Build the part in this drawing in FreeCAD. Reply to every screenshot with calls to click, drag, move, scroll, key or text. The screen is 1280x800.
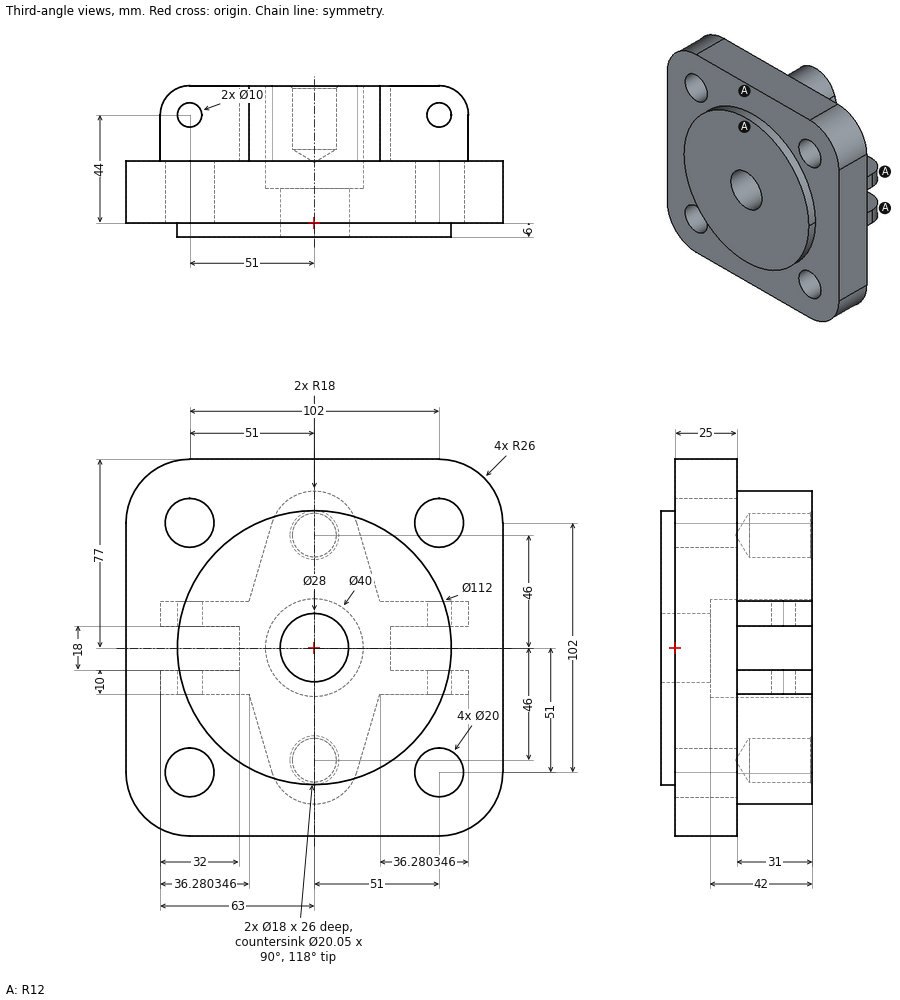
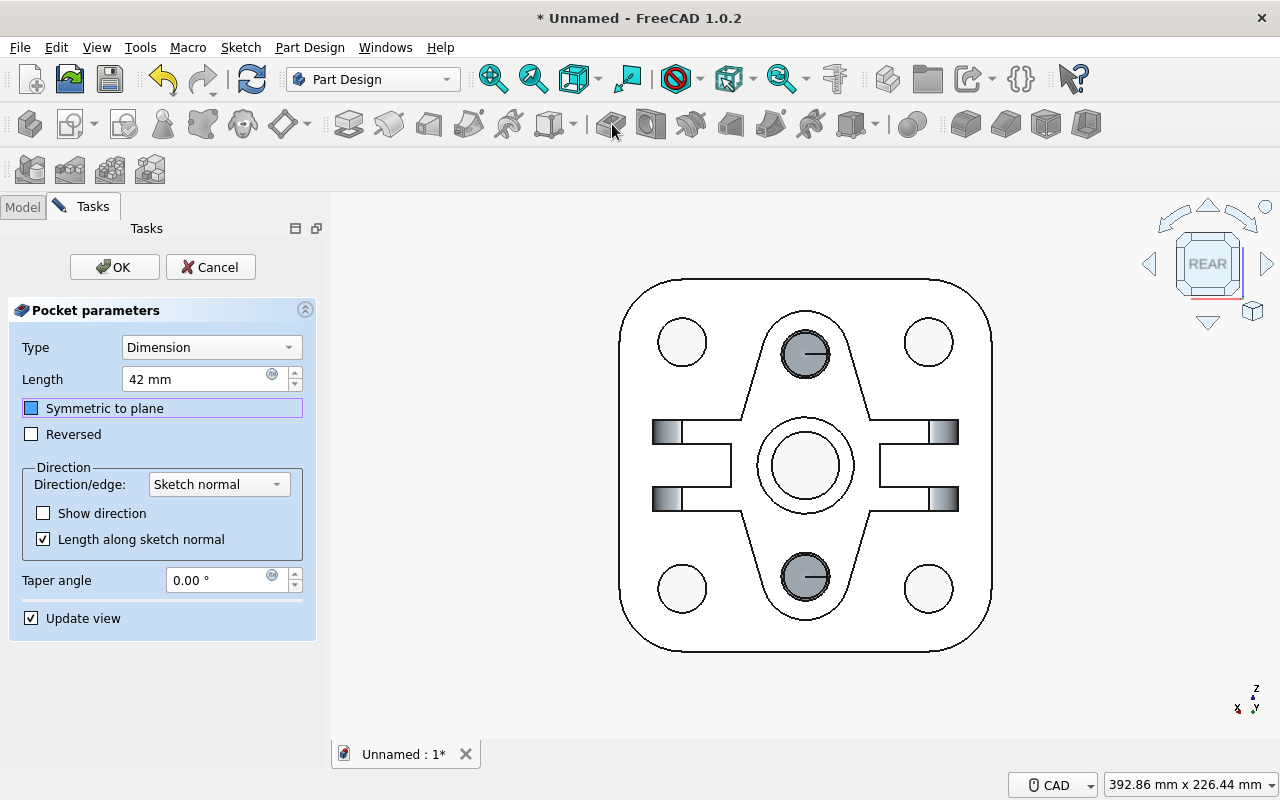
click(115, 267)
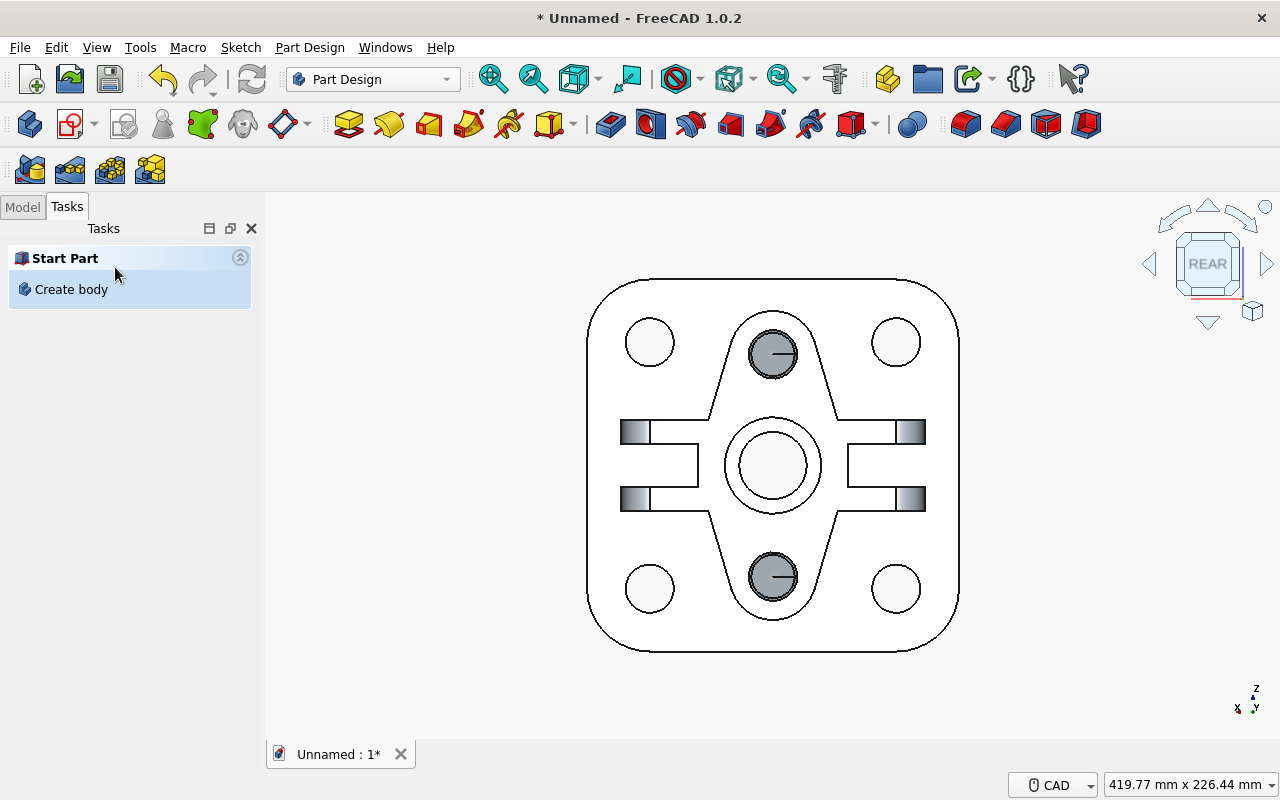
key(0)